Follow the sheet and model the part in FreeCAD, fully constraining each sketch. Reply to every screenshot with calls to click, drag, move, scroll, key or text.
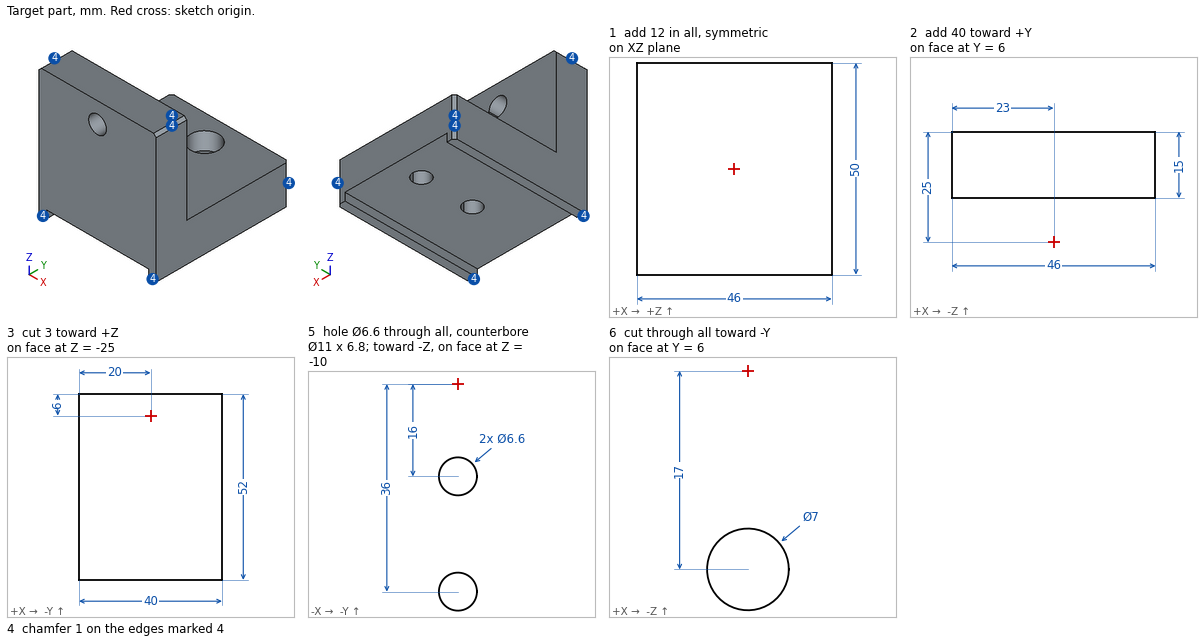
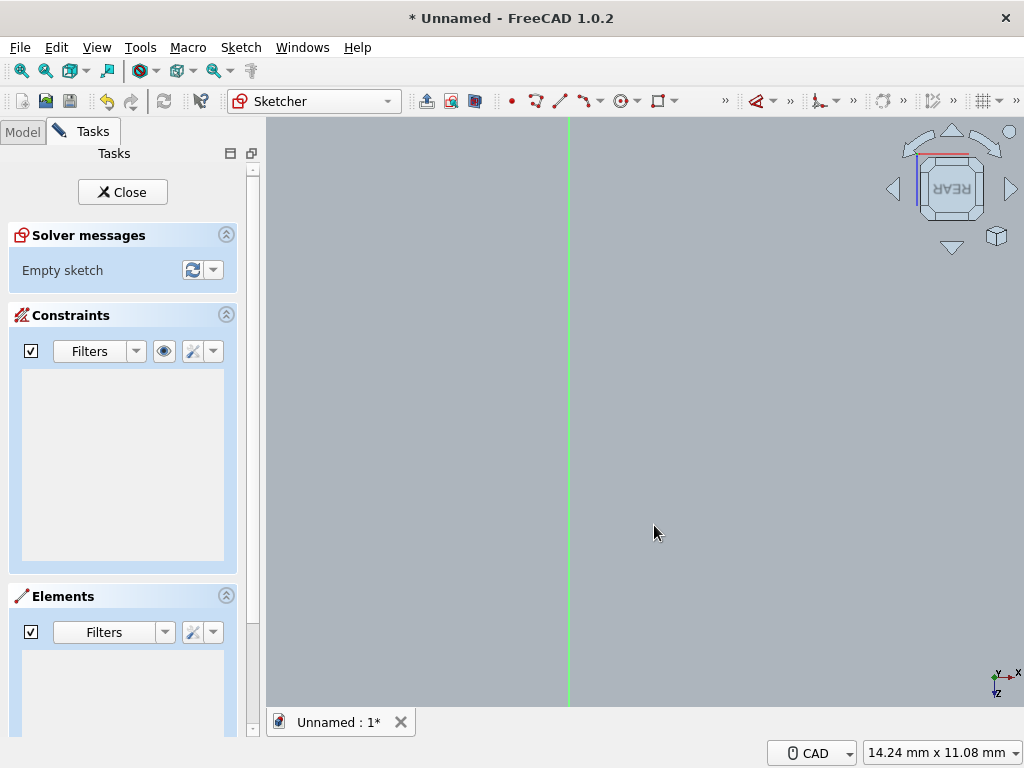
click(622, 102)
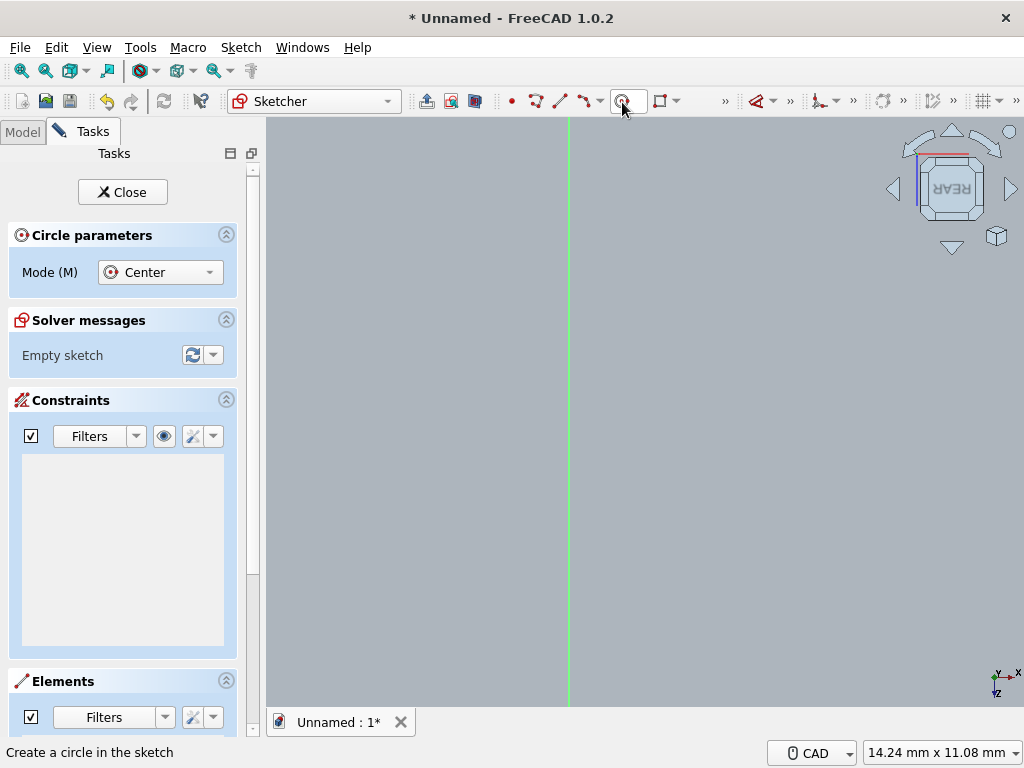
click(569, 405)
move(700, 273)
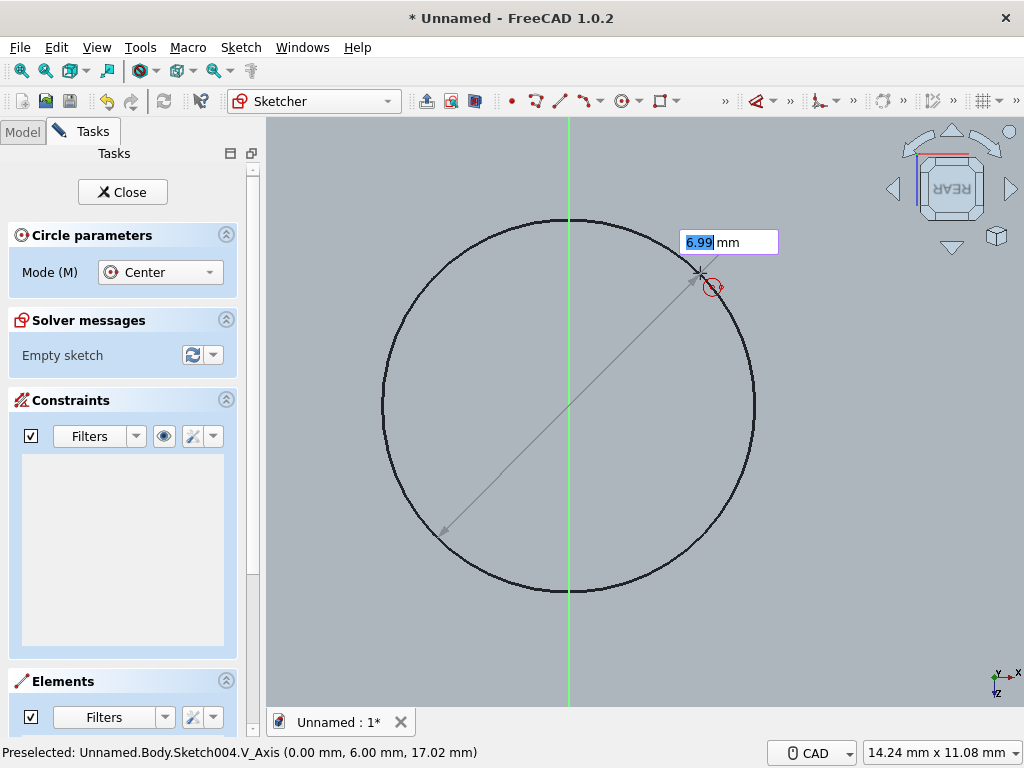
text(7)
key(Return)
key(Escape)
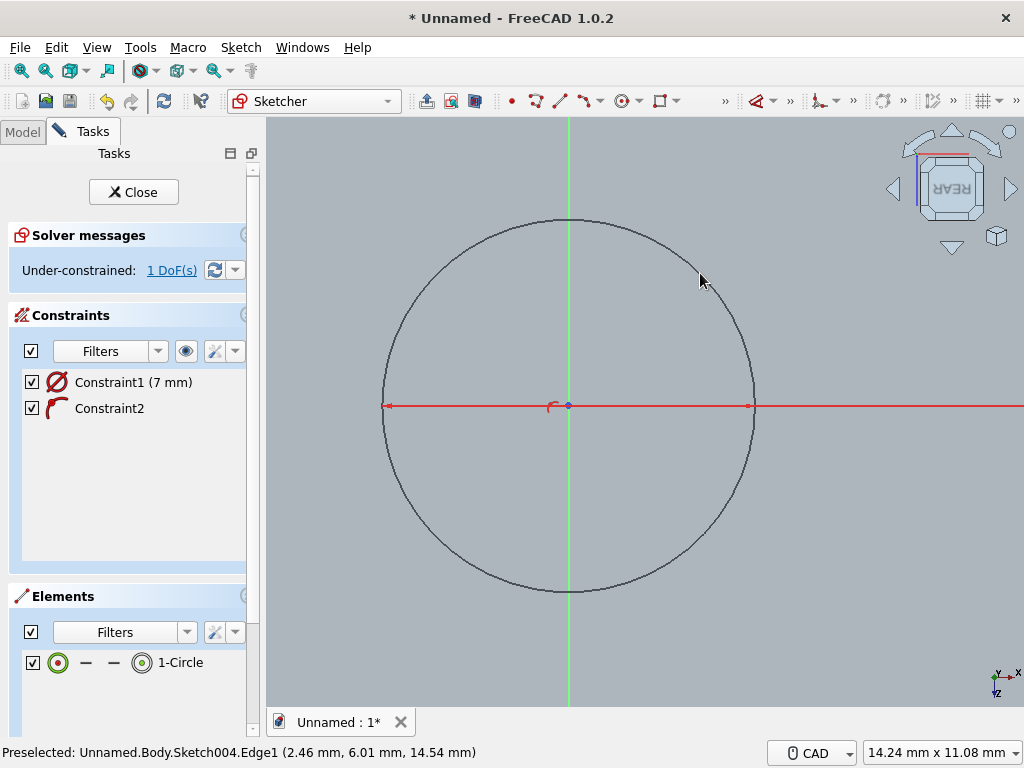
click(756, 102)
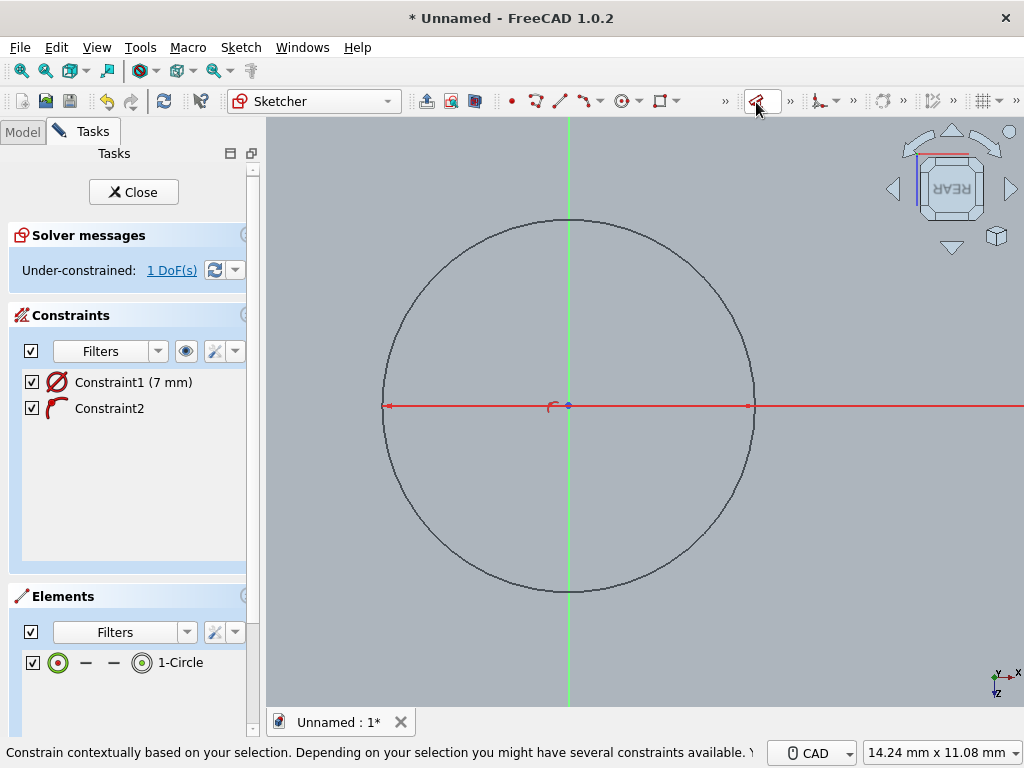
click(569, 406)
click(603, 276)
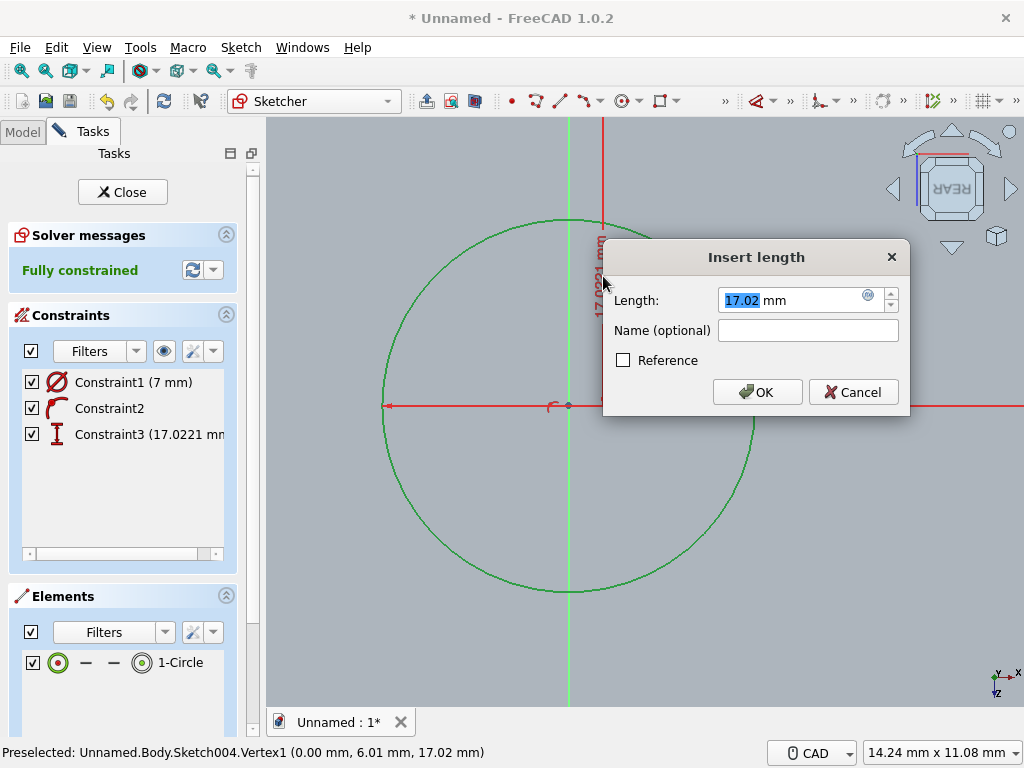
text(17)
key(Return)
key(Escape)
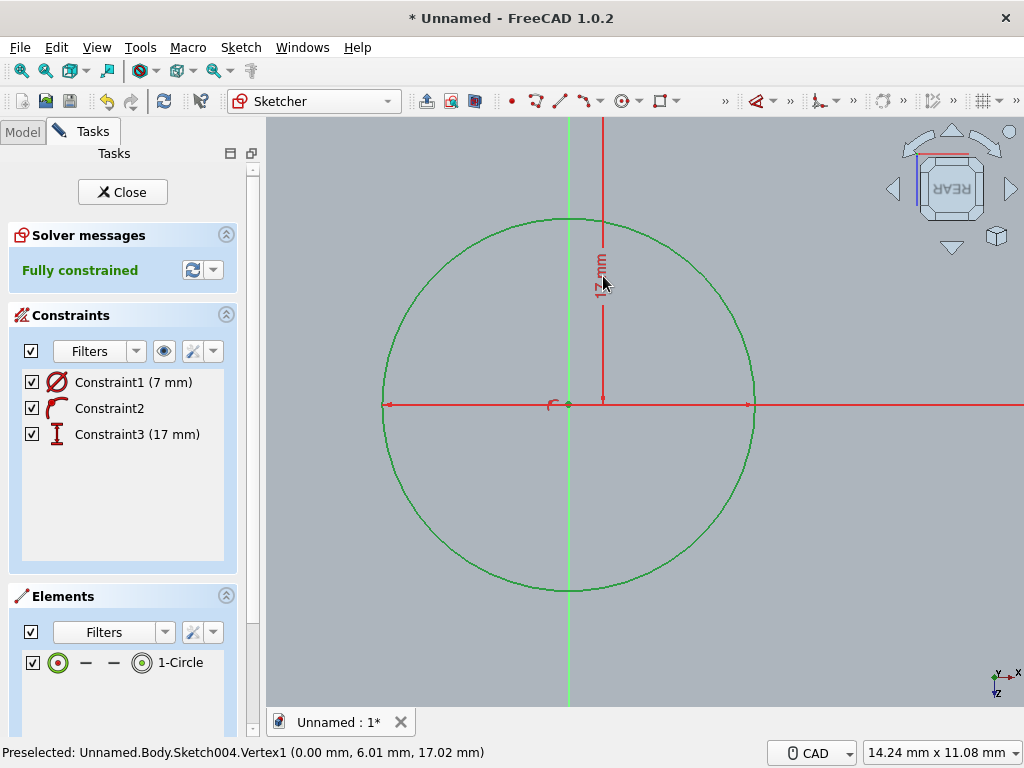
click(123, 192)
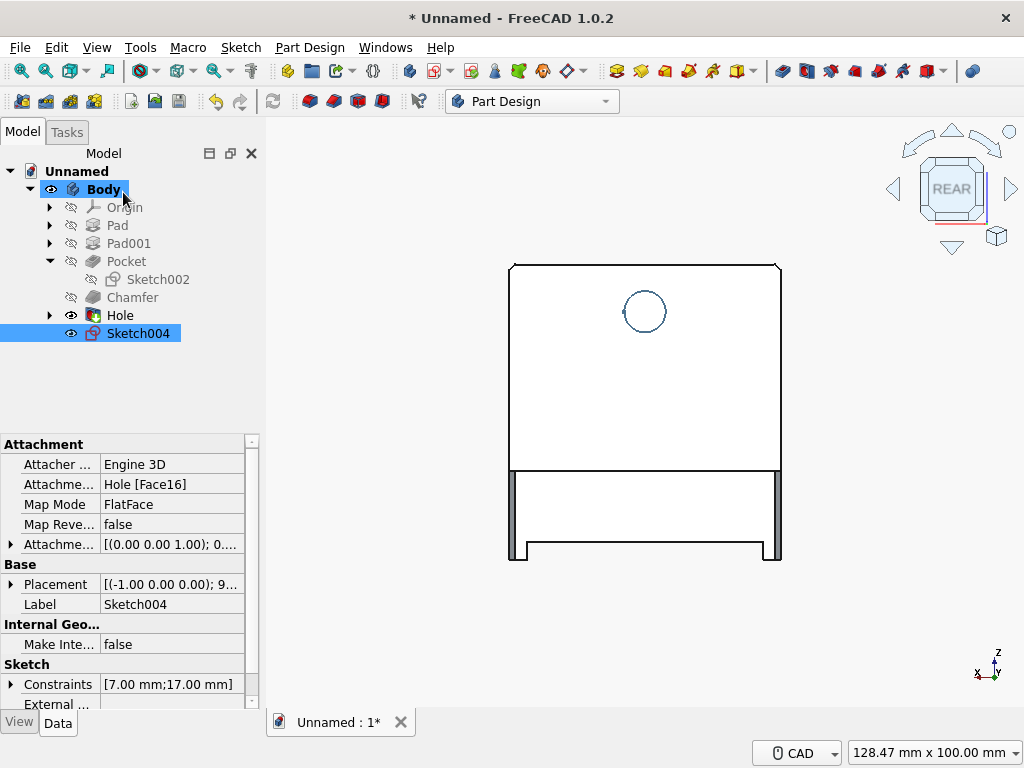
click(784, 72)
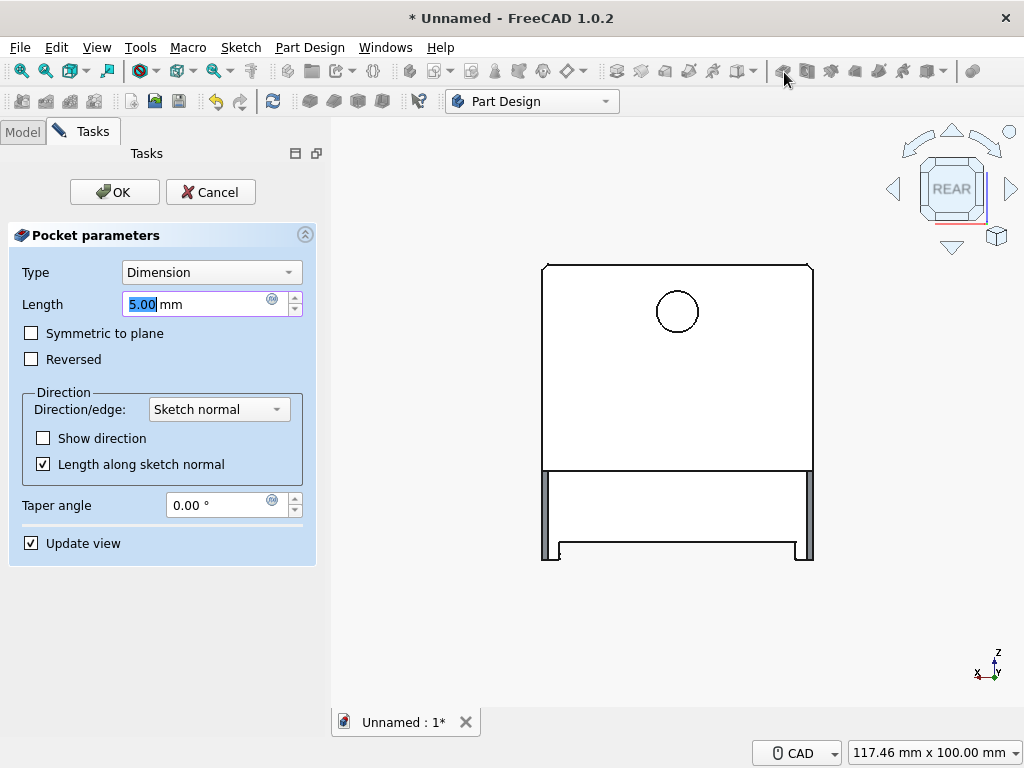
click(212, 272)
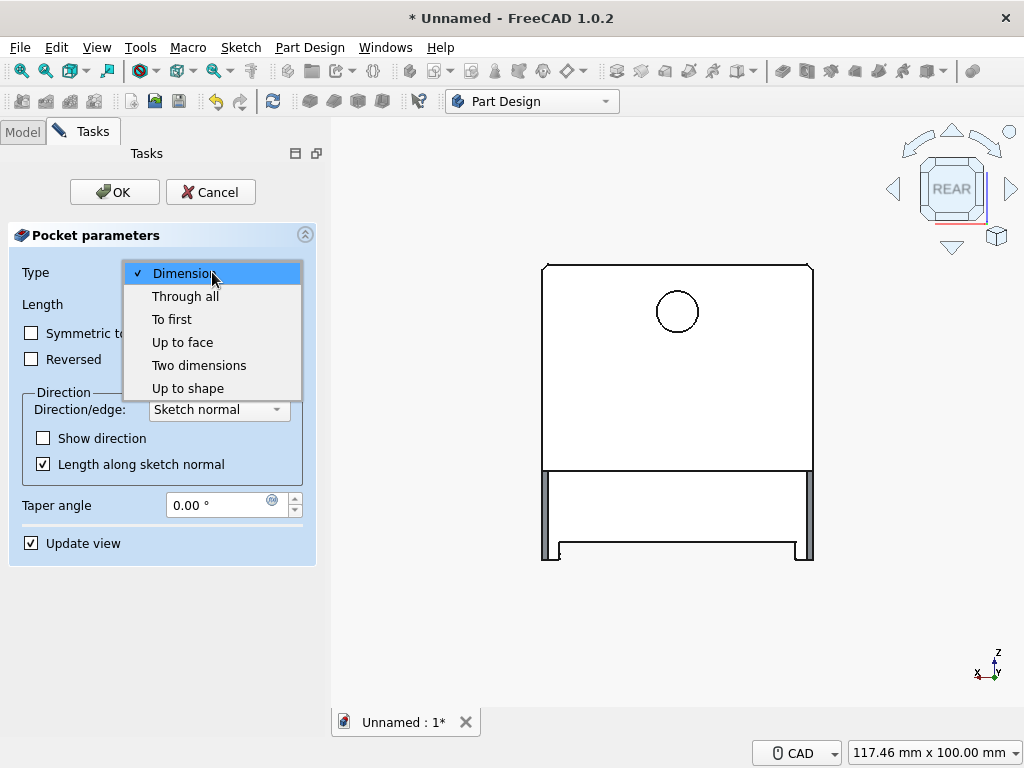
click(212, 296)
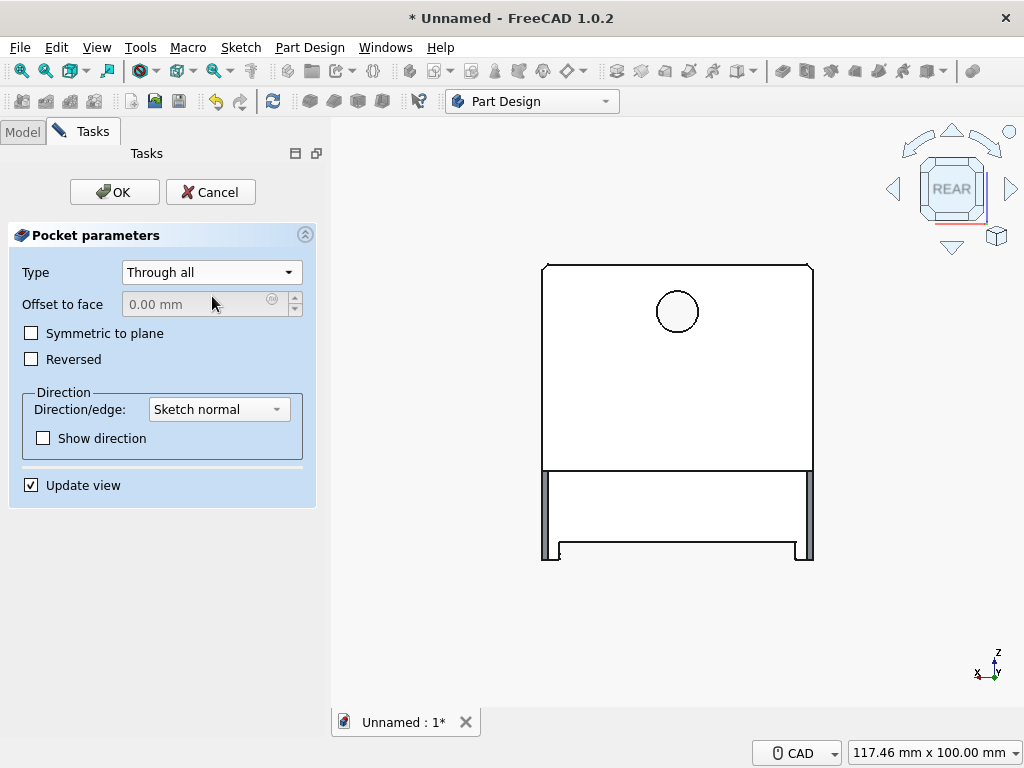
click(115, 192)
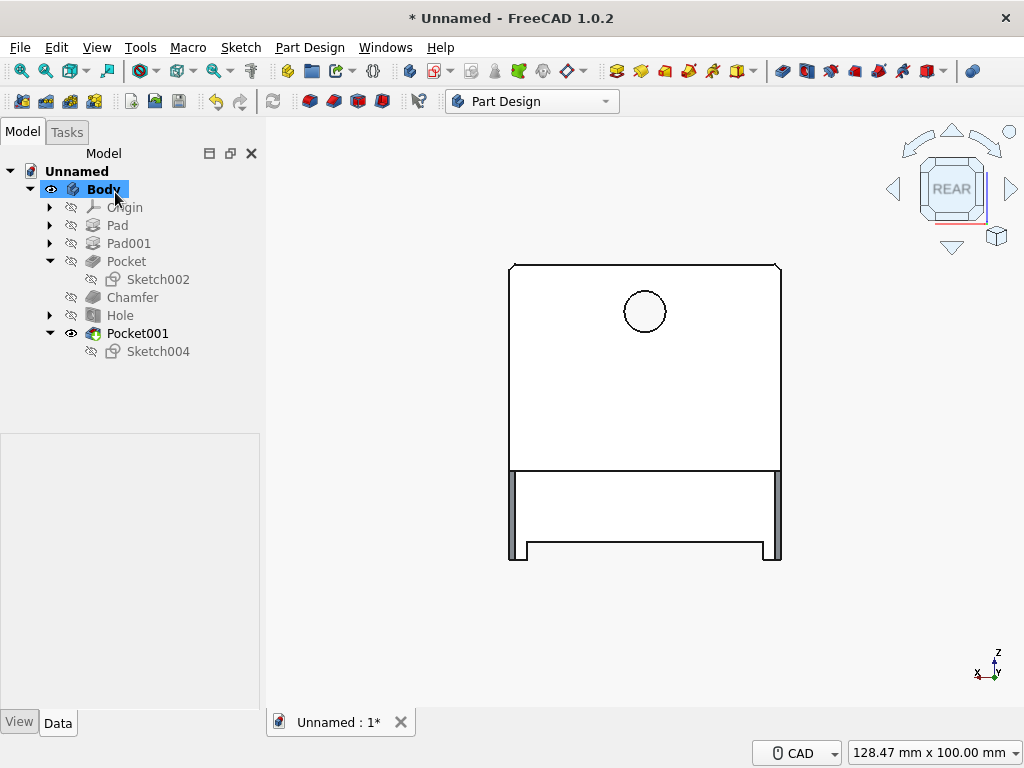
key(0)